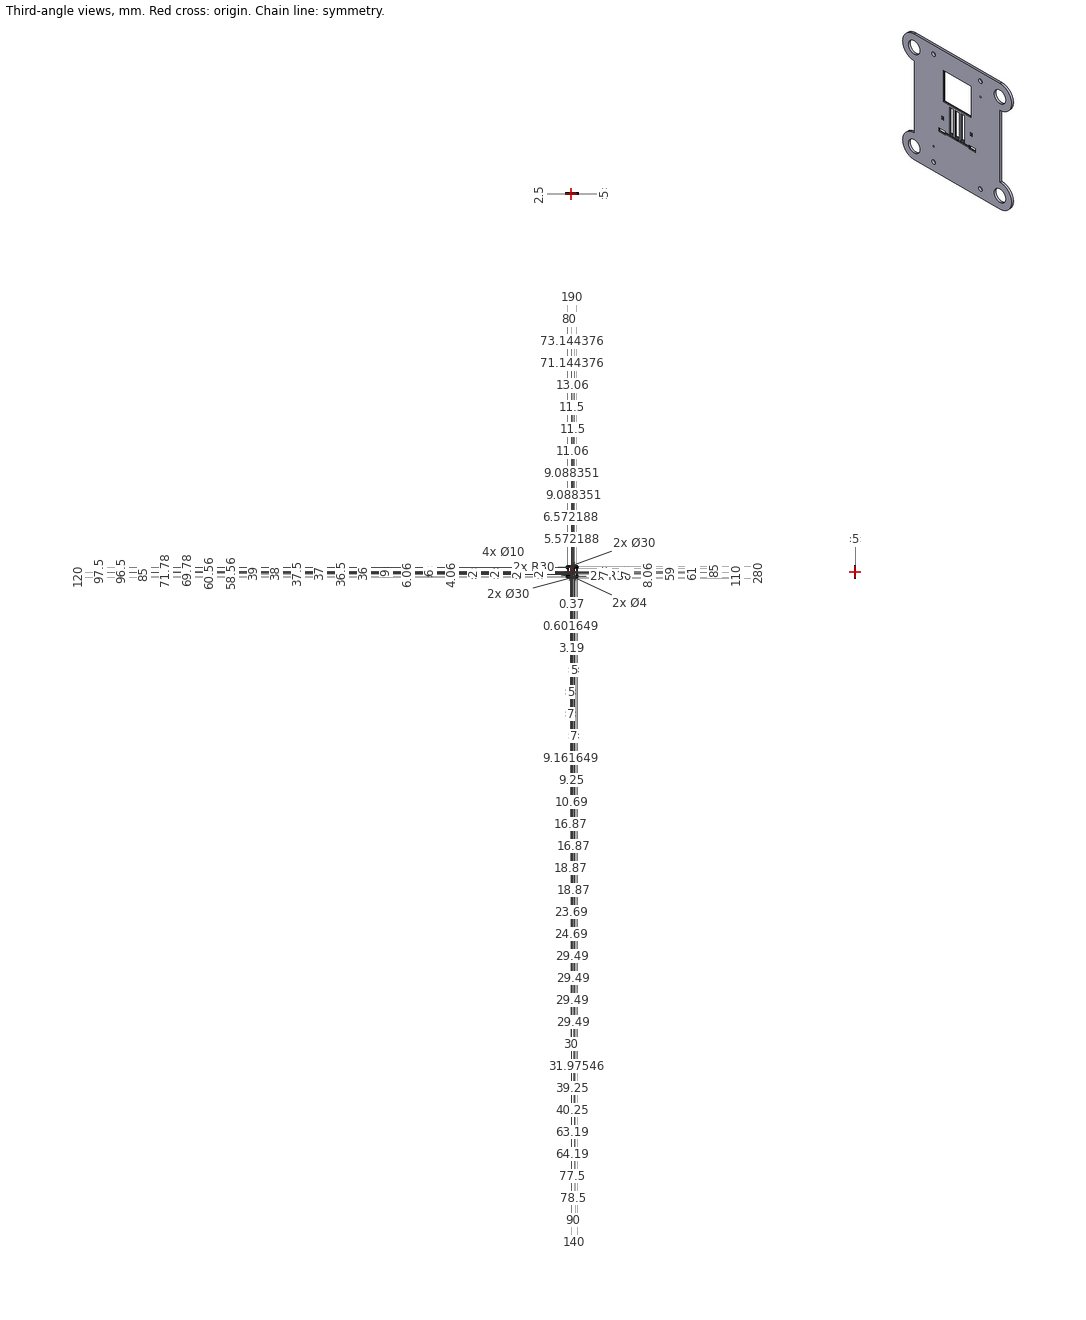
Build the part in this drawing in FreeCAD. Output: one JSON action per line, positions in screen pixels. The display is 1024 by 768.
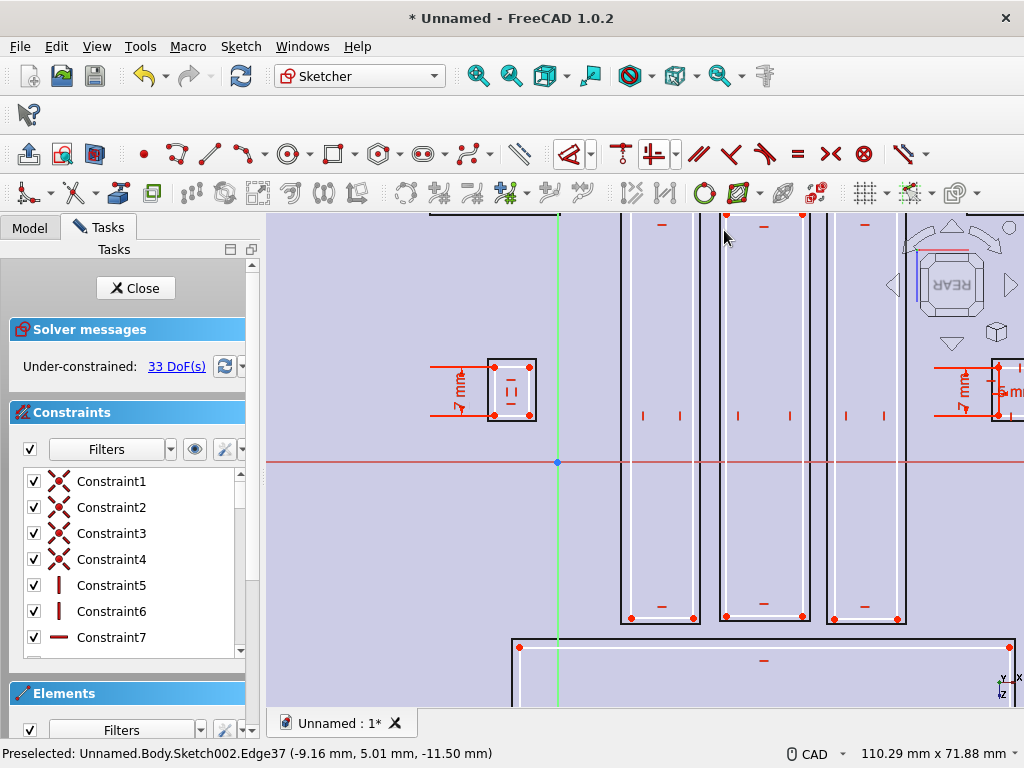
{"action": "scroll", "coordinate": [505, 416], "scroll_direction": "up", "scroll_amount": 2}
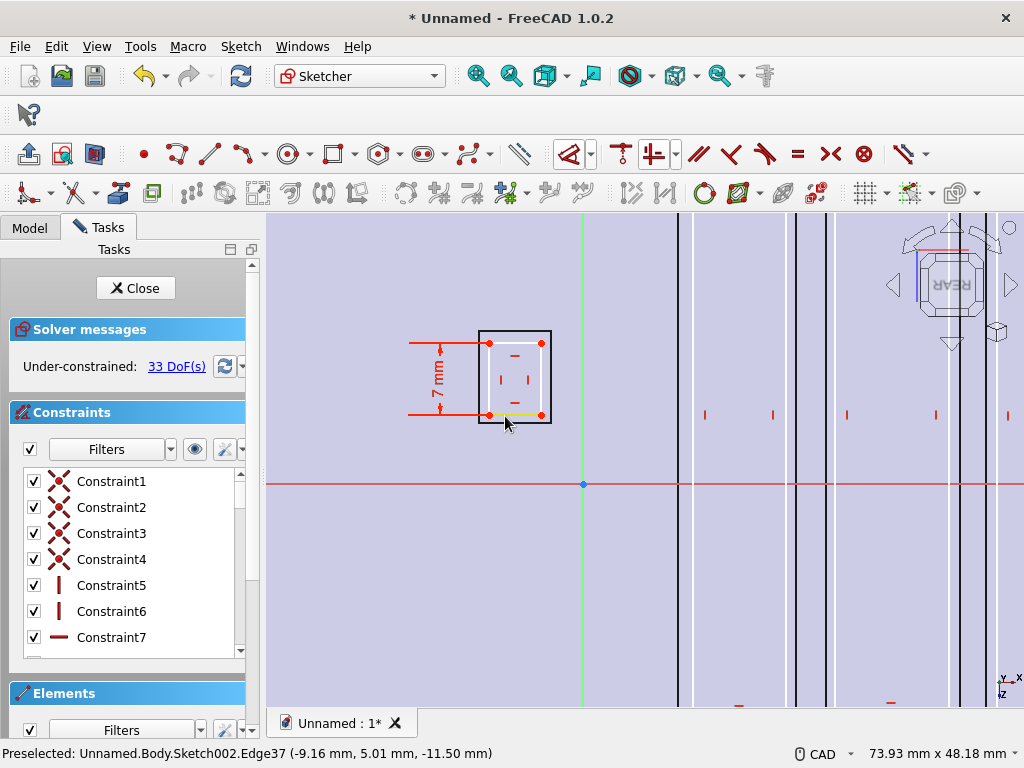
{"action": "left_click", "coordinate": [505, 415]}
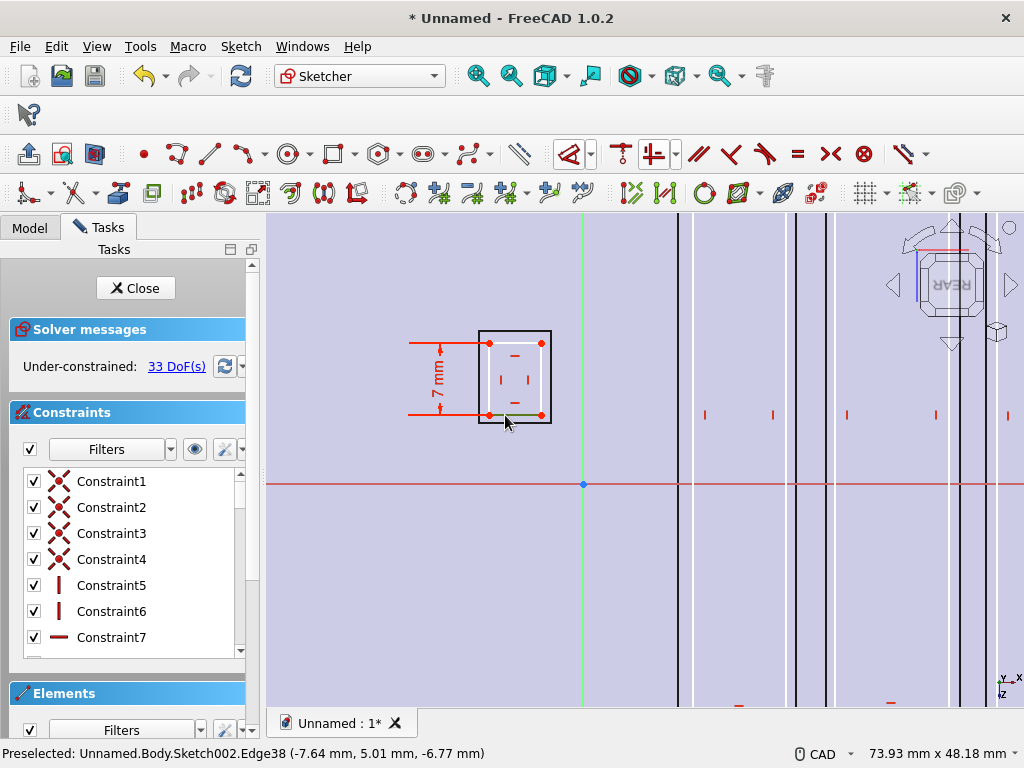
{"action": "key", "text": "l"}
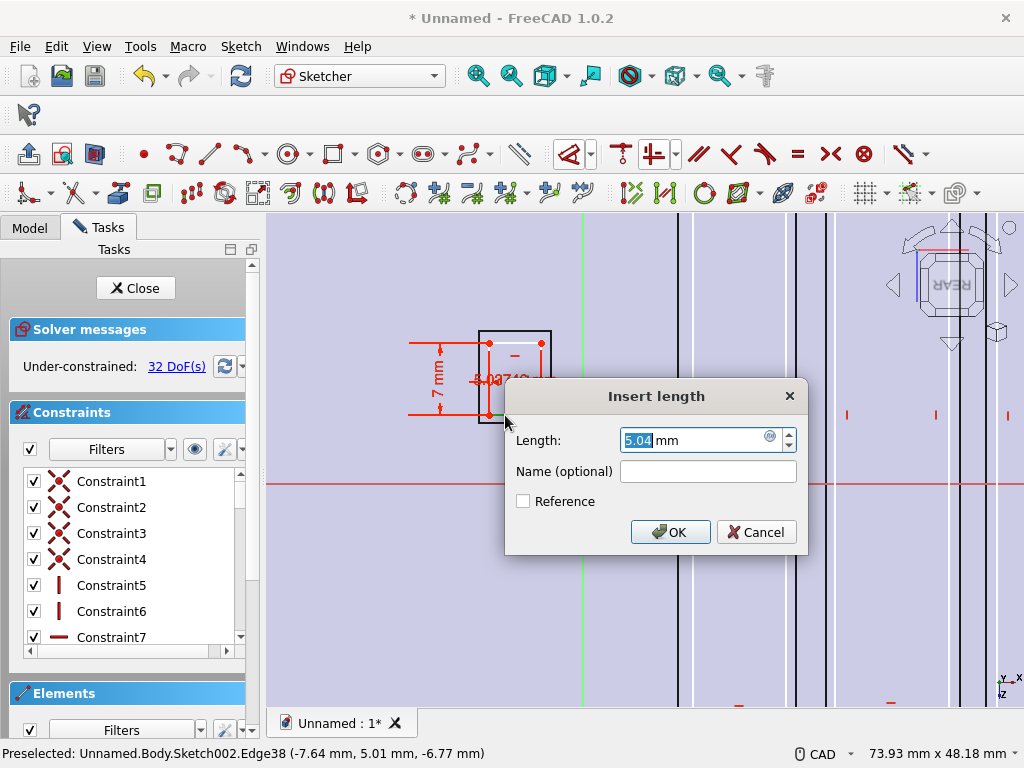
{"action": "type", "text": "5"}
{"action": "key", "text": "Return"}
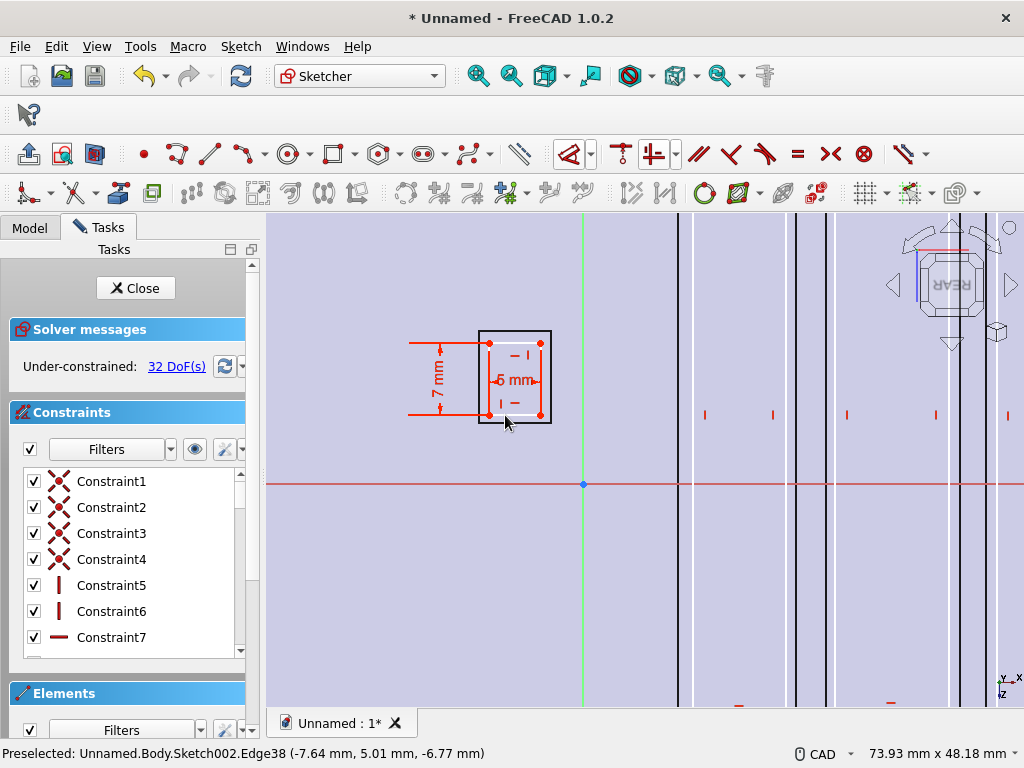
{"action": "scroll", "coordinate": [497, 387], "scroll_direction": "down", "scroll_amount": 8}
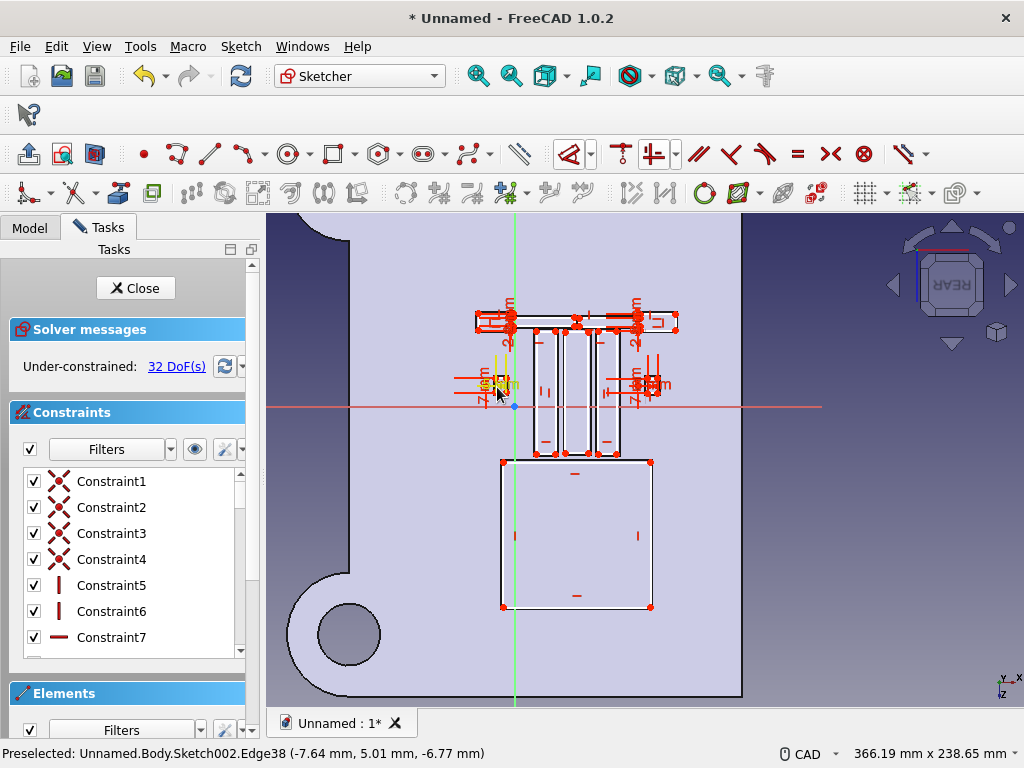
{"action": "scroll", "coordinate": [598, 369], "scroll_direction": "up", "scroll_amount": 2}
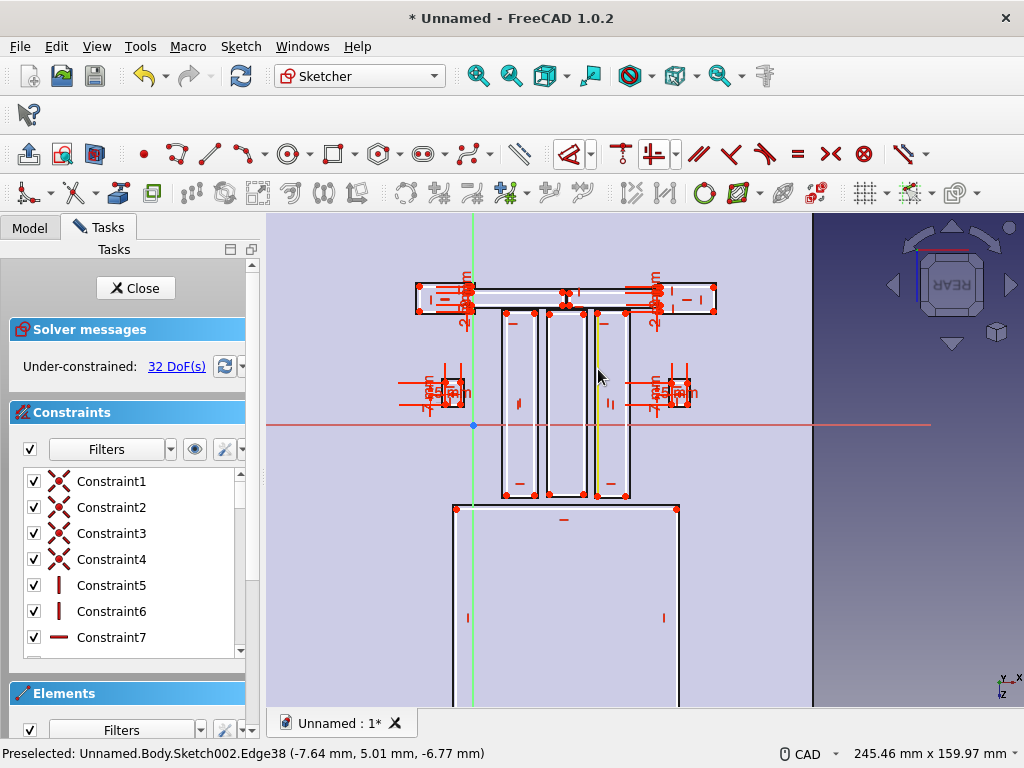
{"action": "left_click", "coordinate": [598, 368]}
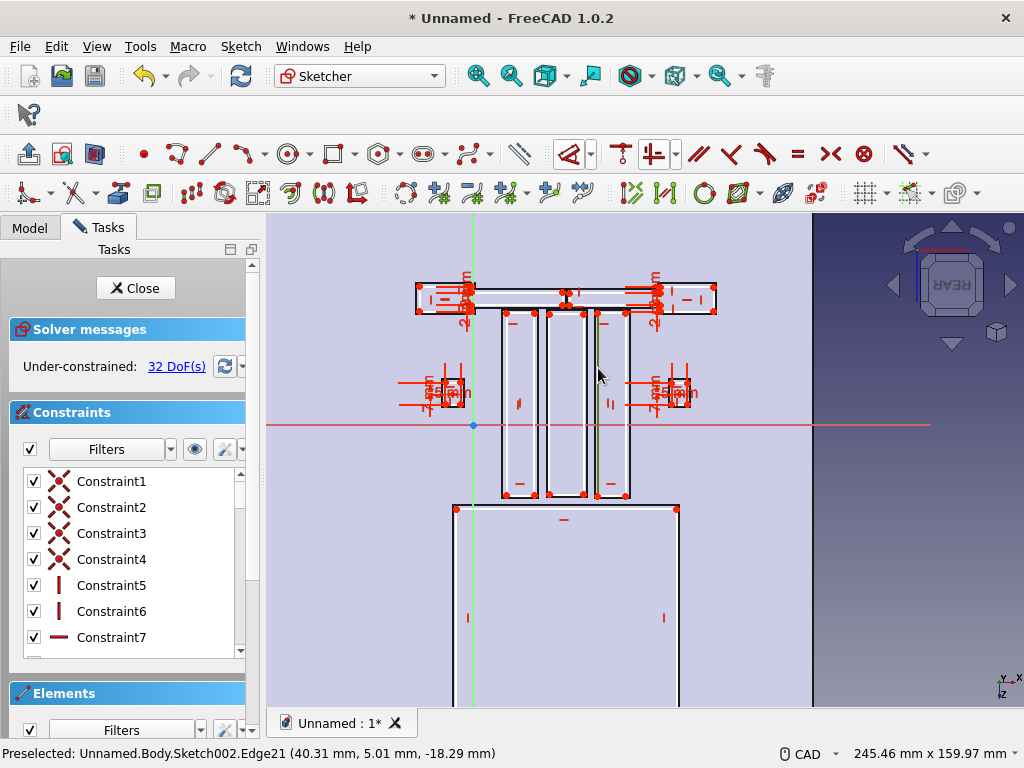
{"action": "key", "text": "i"}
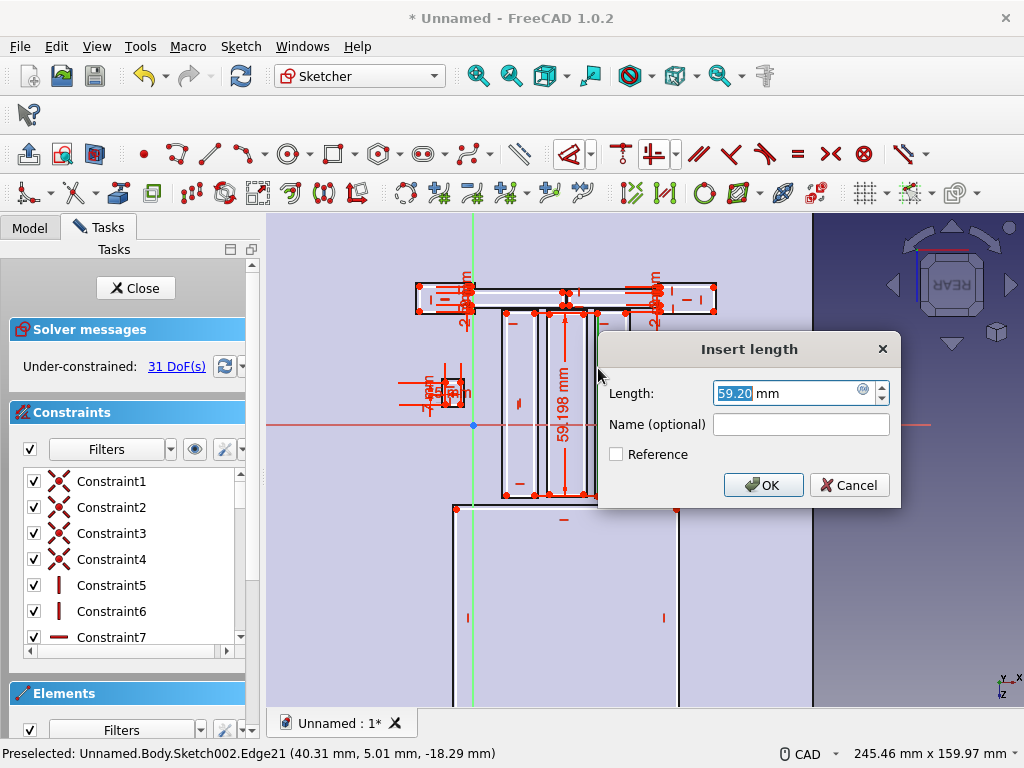
{"action": "type", "text": "59"}
{"action": "key", "text": "Return"}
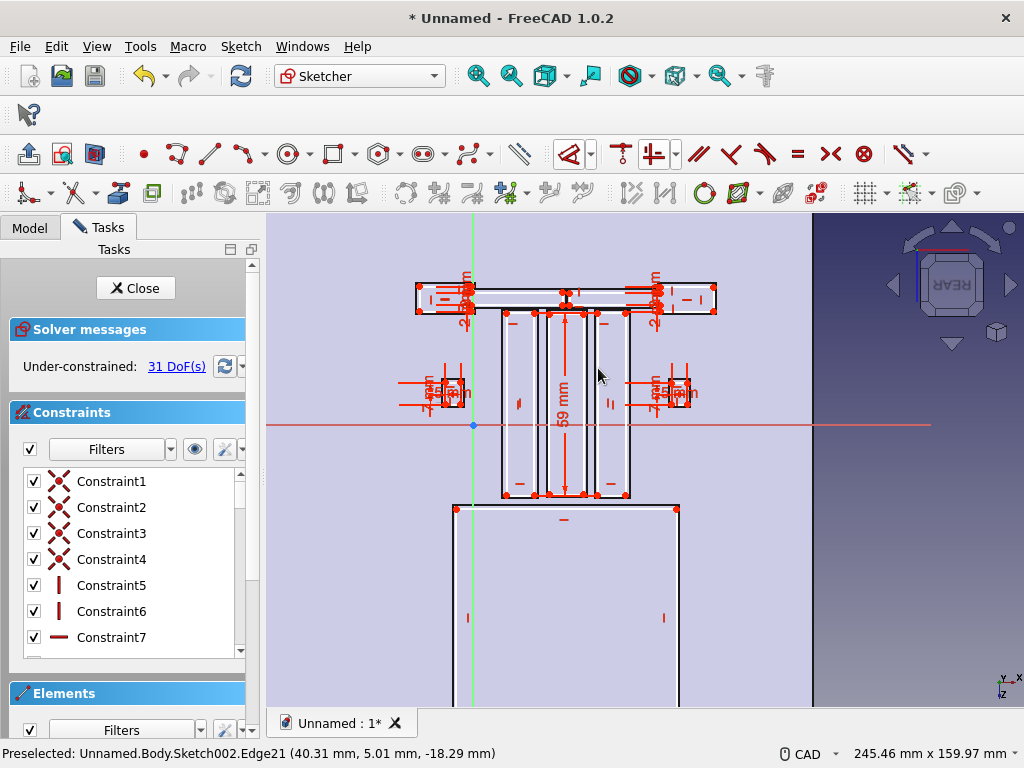
{"action": "left_click", "coordinate": [507, 368]}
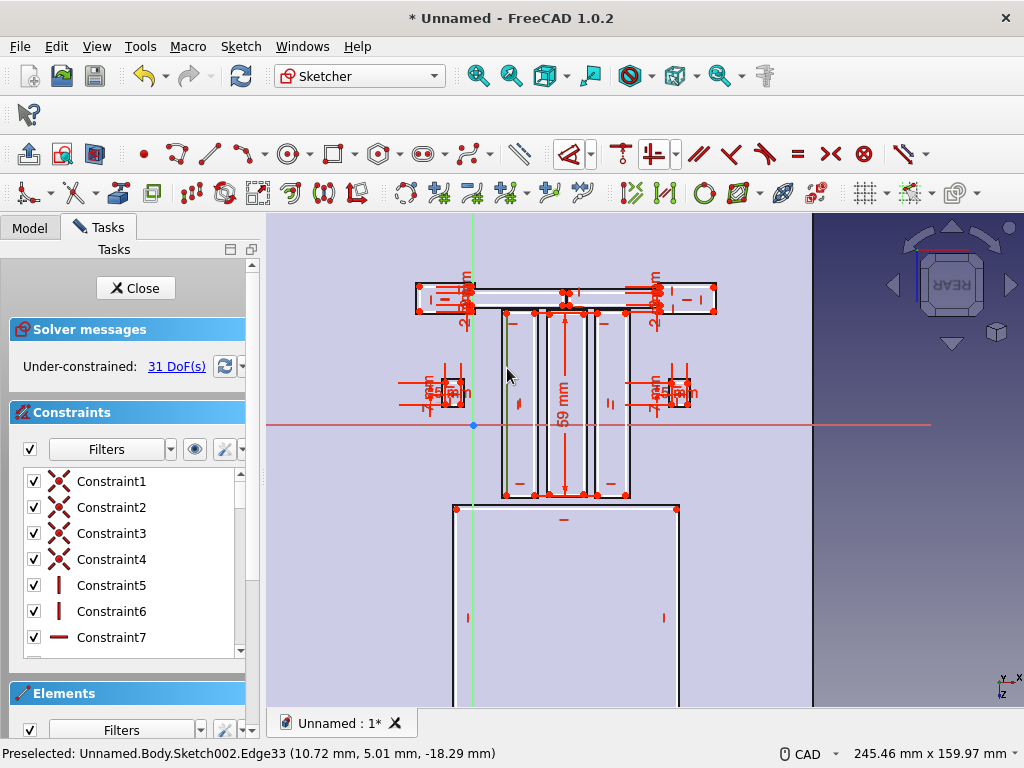
{"action": "left_click", "coordinate": [590, 154]}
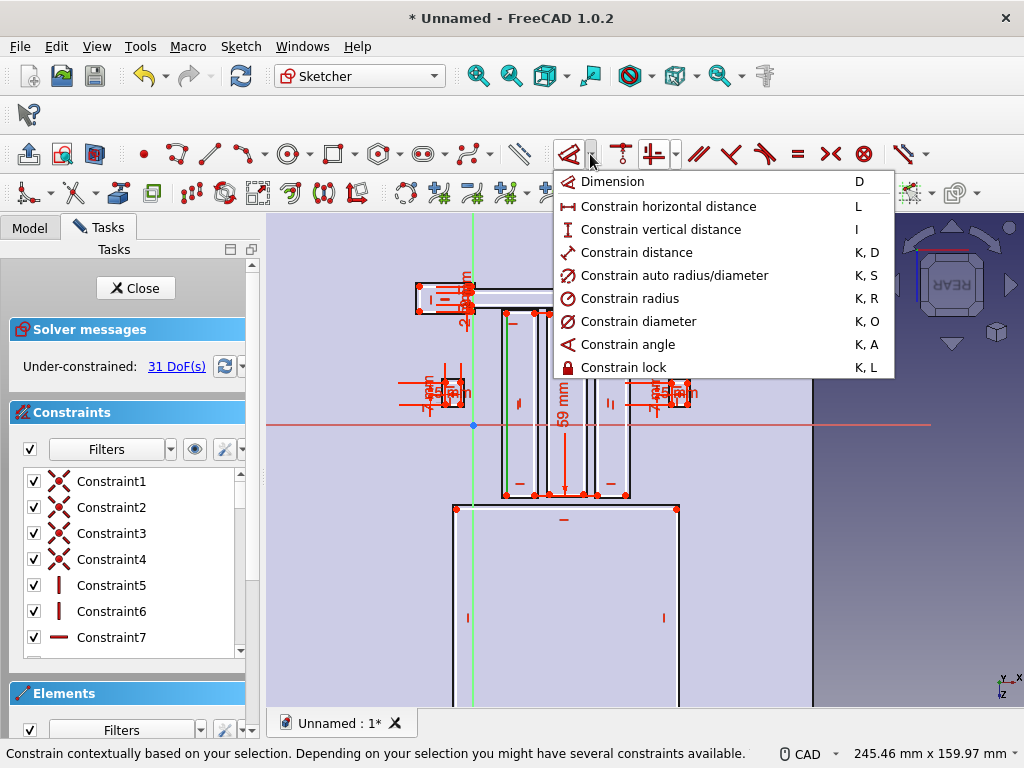
{"action": "left_click", "coordinate": [724, 230]}